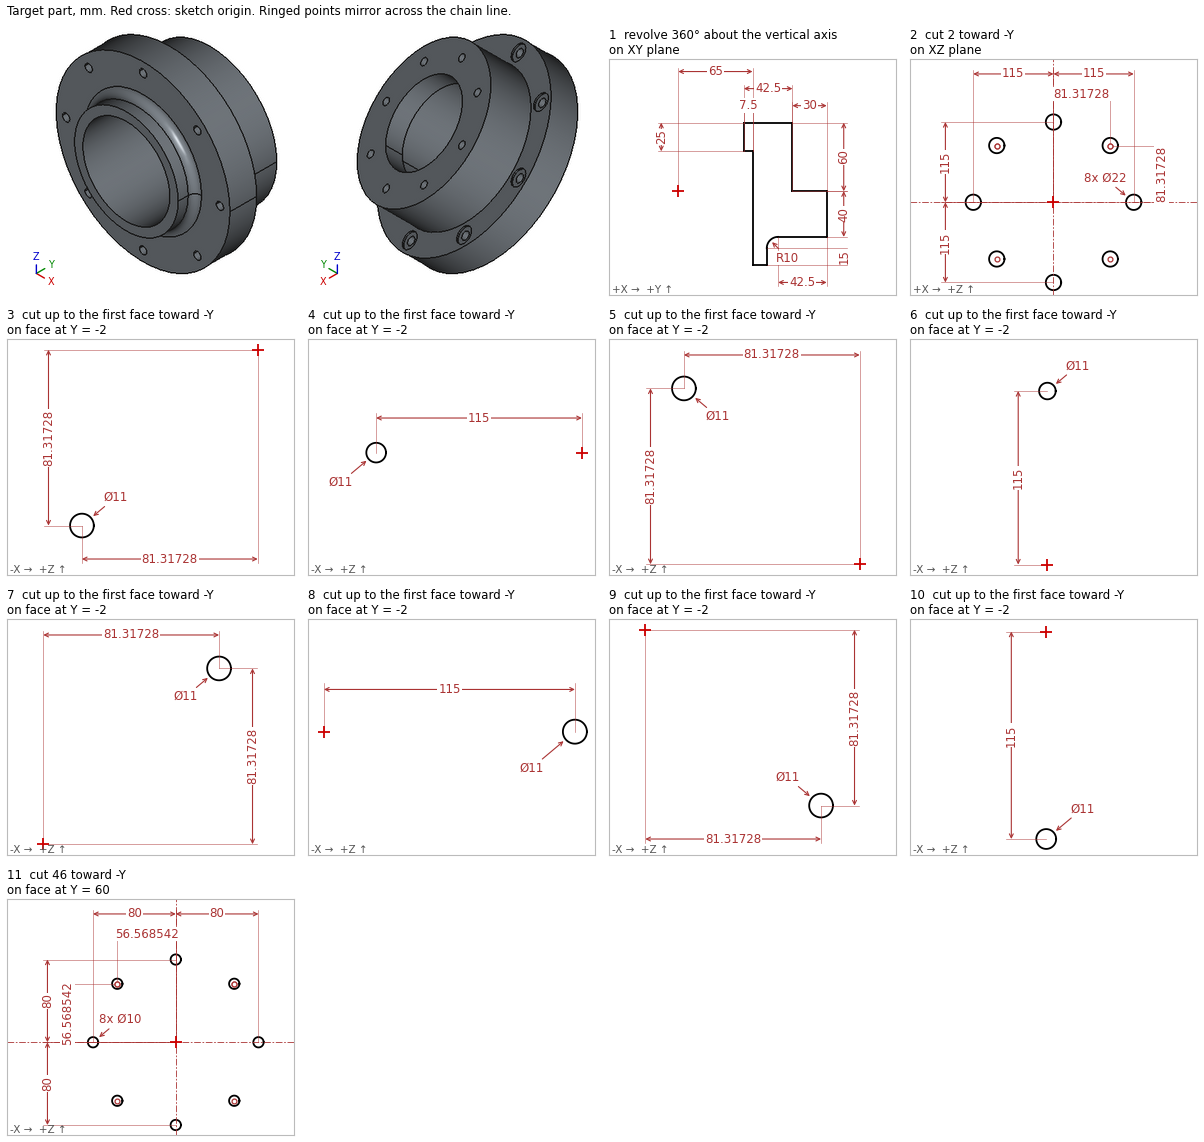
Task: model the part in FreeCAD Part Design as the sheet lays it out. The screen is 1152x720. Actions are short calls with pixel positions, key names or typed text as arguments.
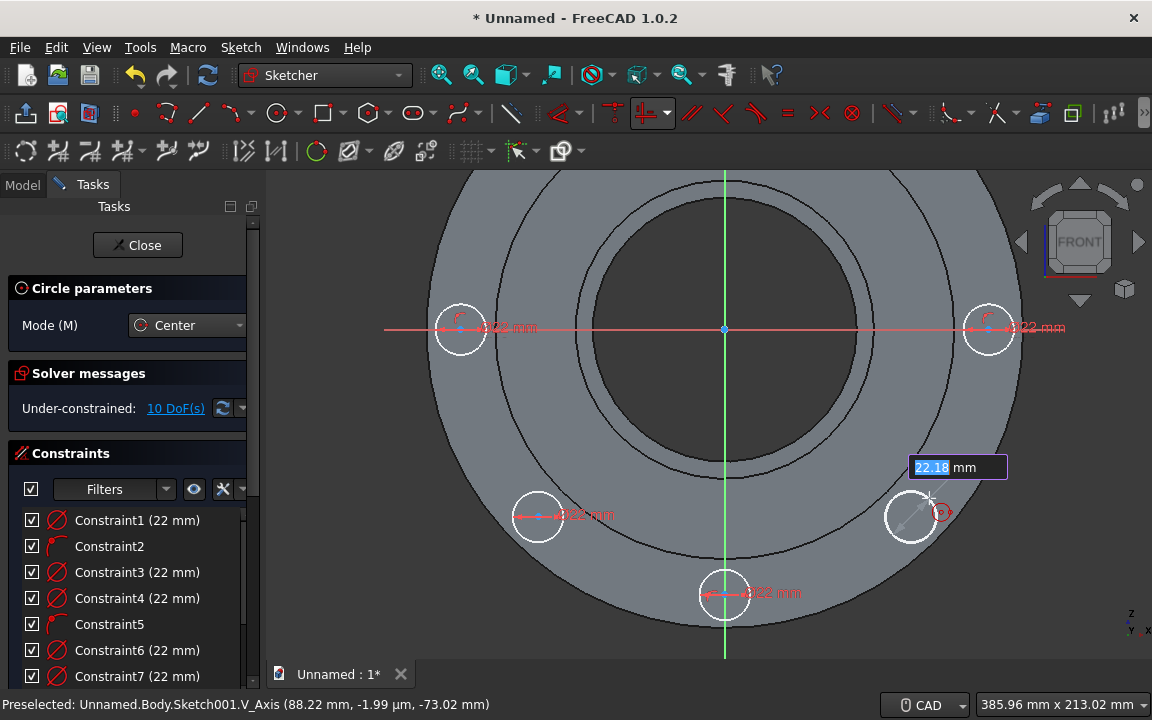
text(22)
key(Return)
key(Escape)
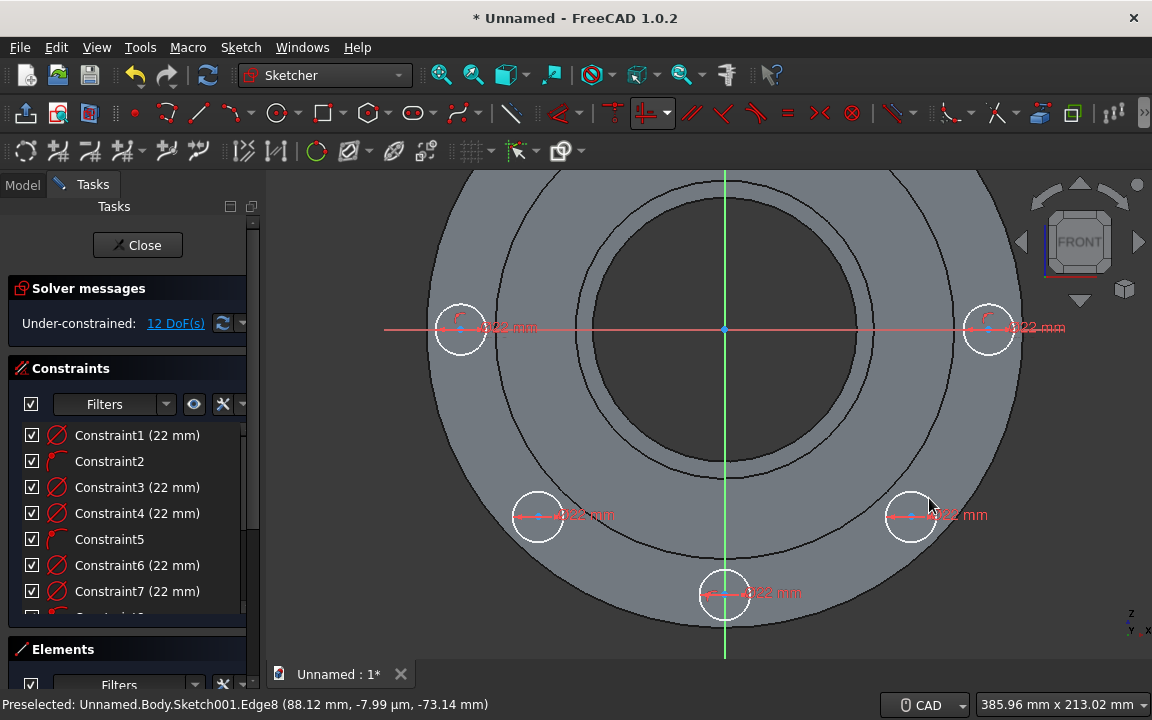
scroll(538, 518, down, 3)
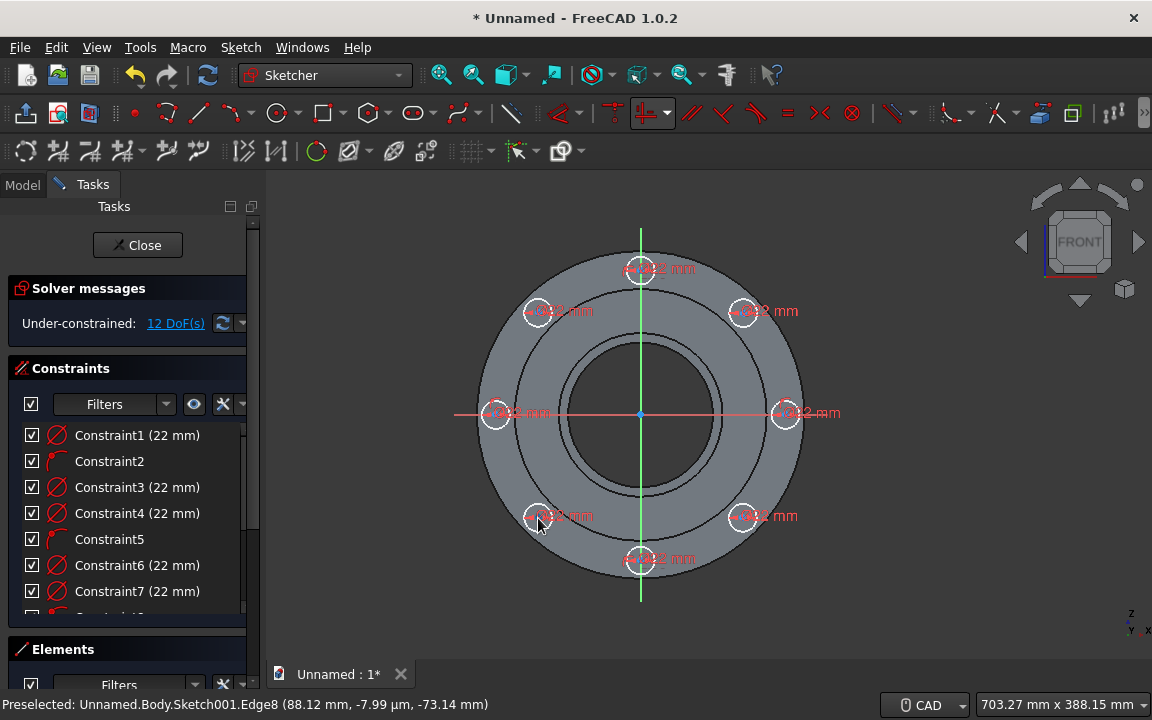
click(743, 313)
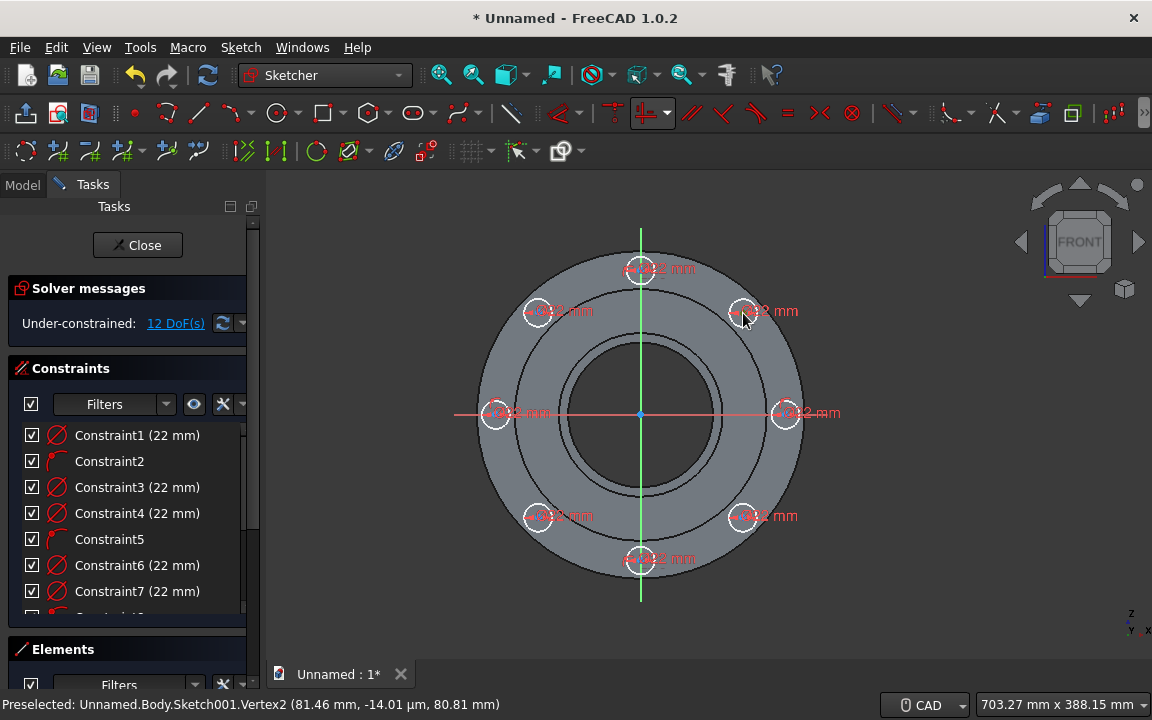
click(538, 313)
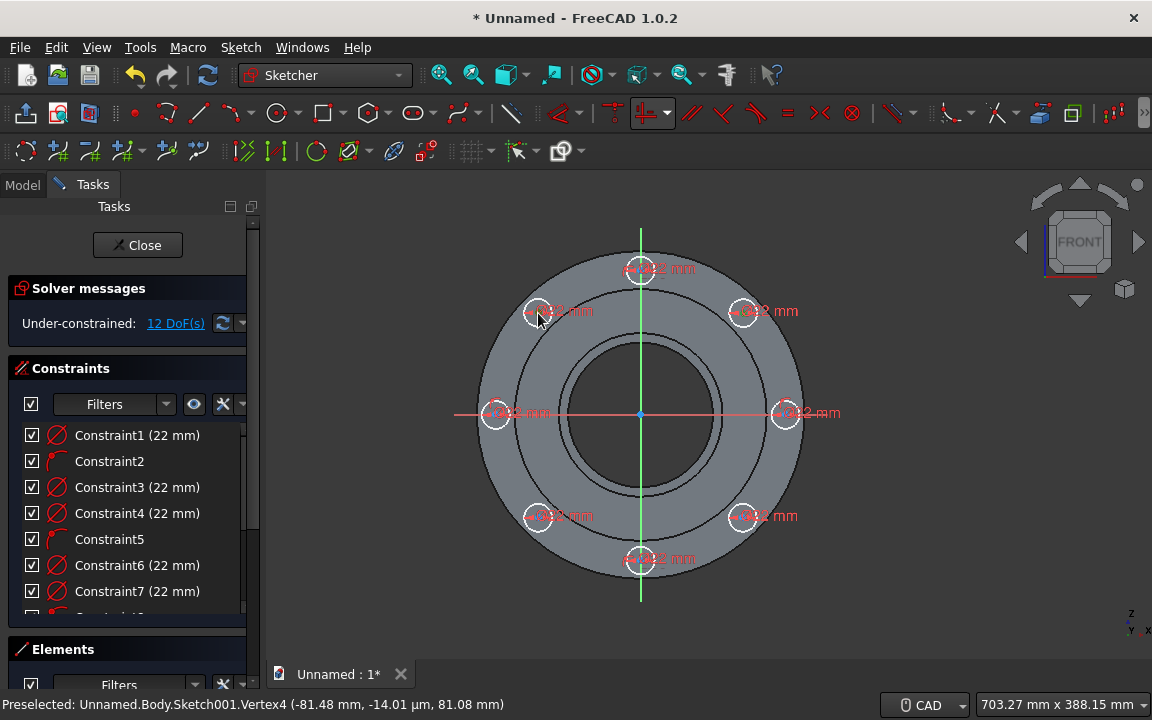
click(641, 507)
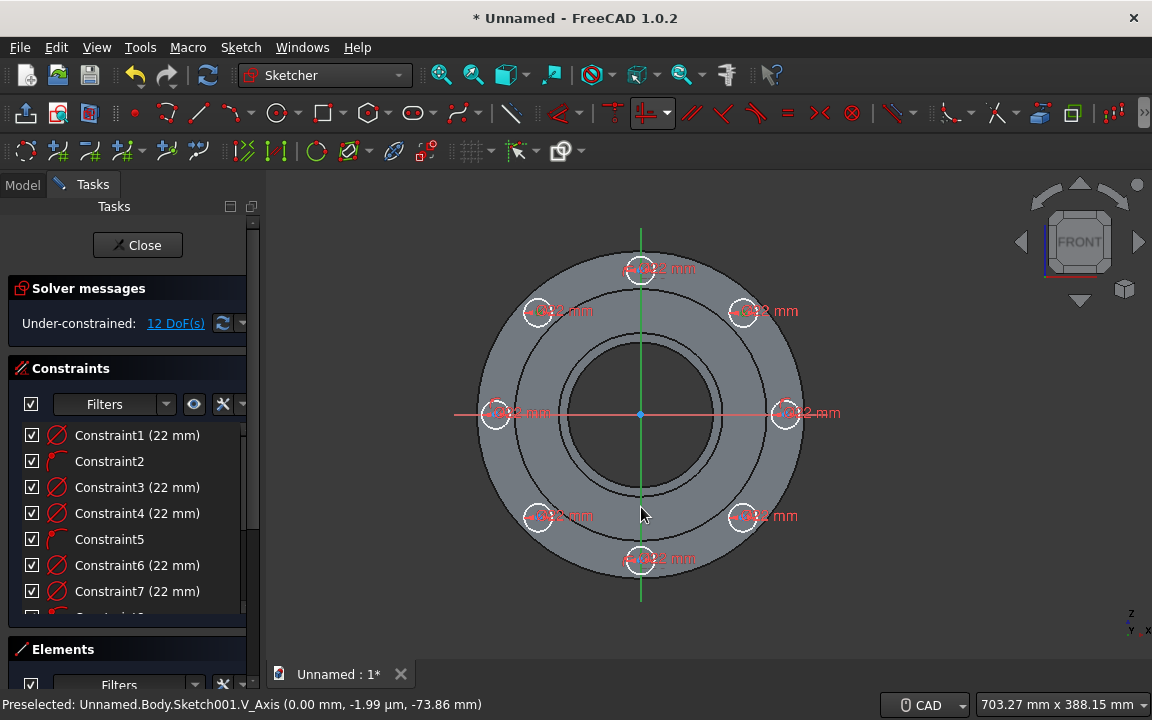
key(s)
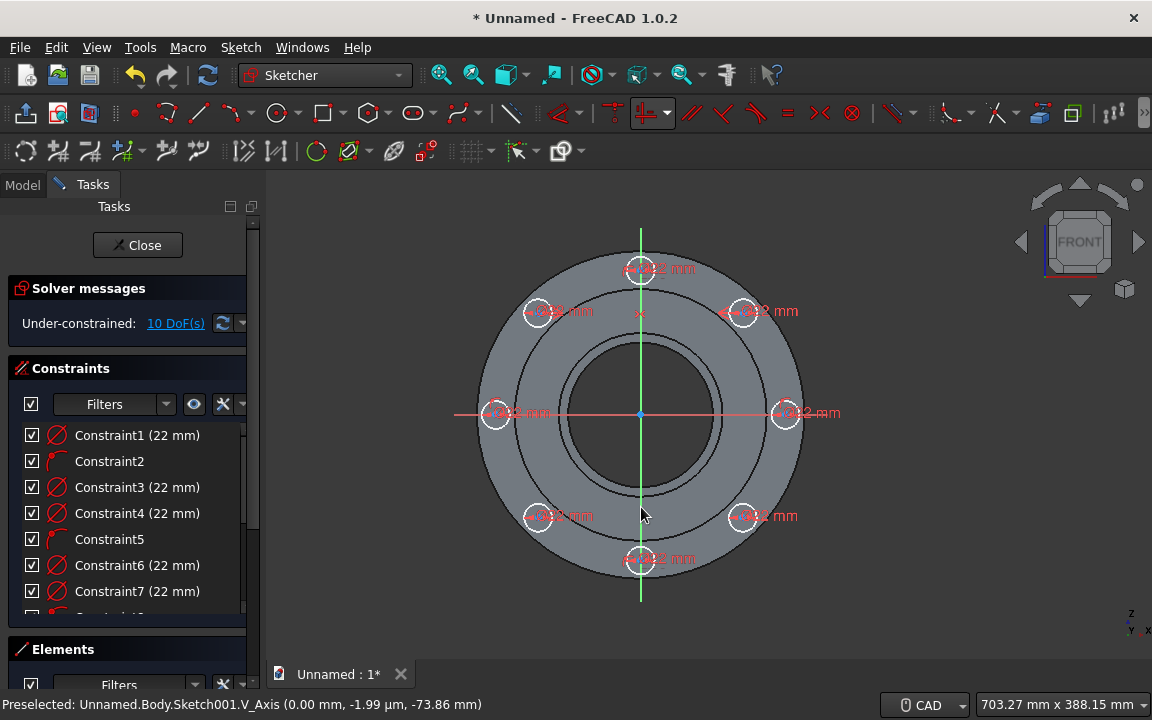
click(538, 313)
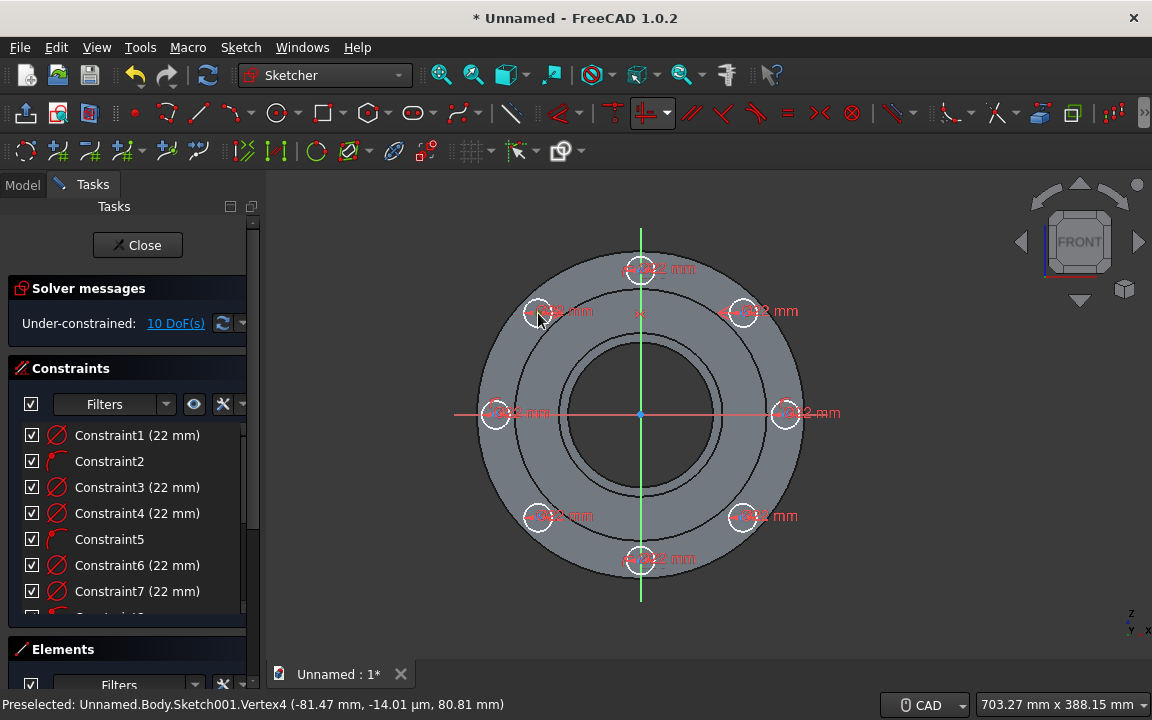
click(538, 518)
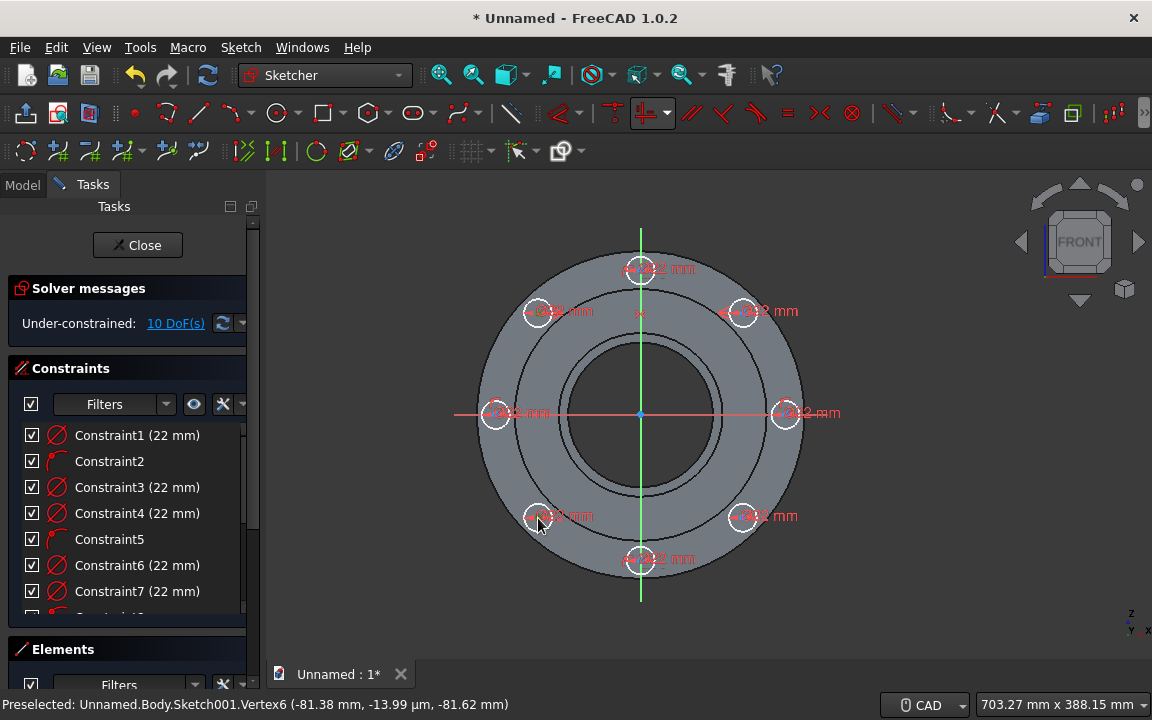
click(591, 415)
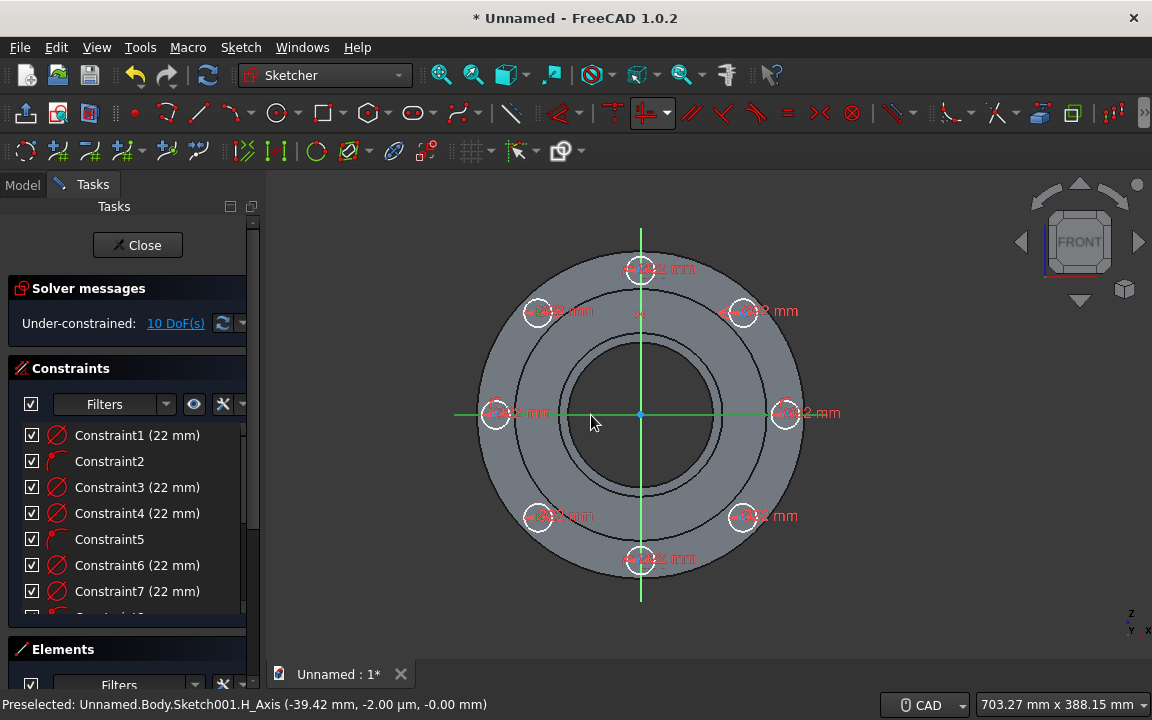
click(820, 114)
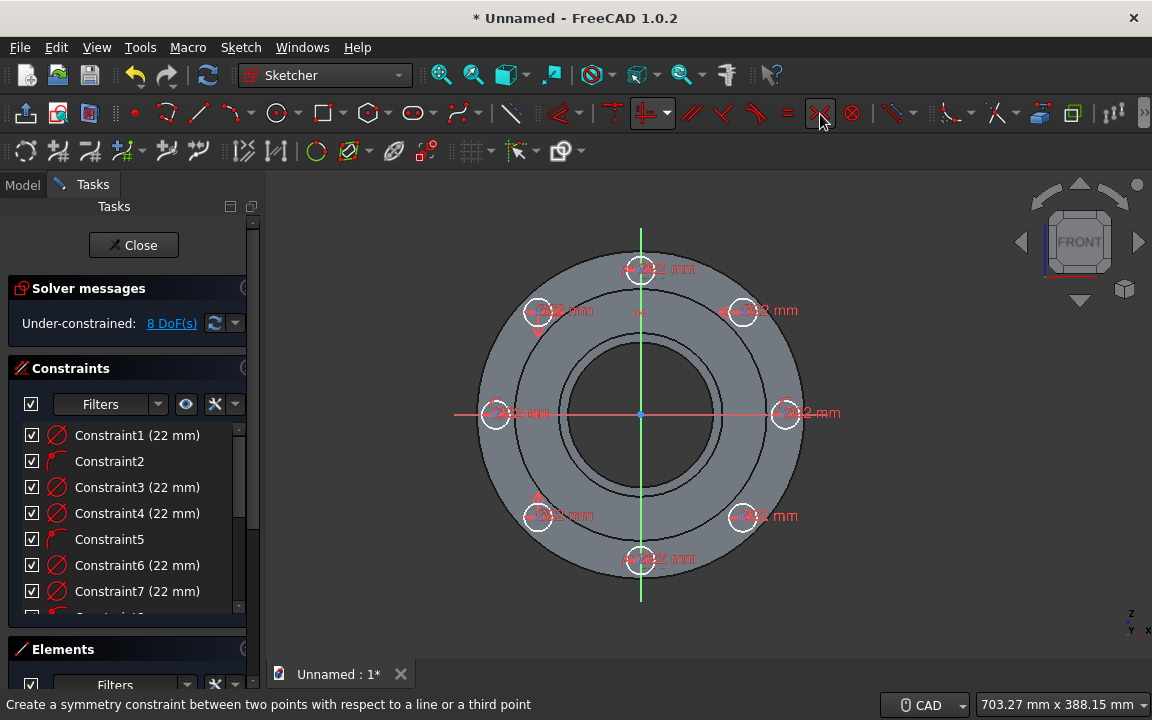
click(743, 312)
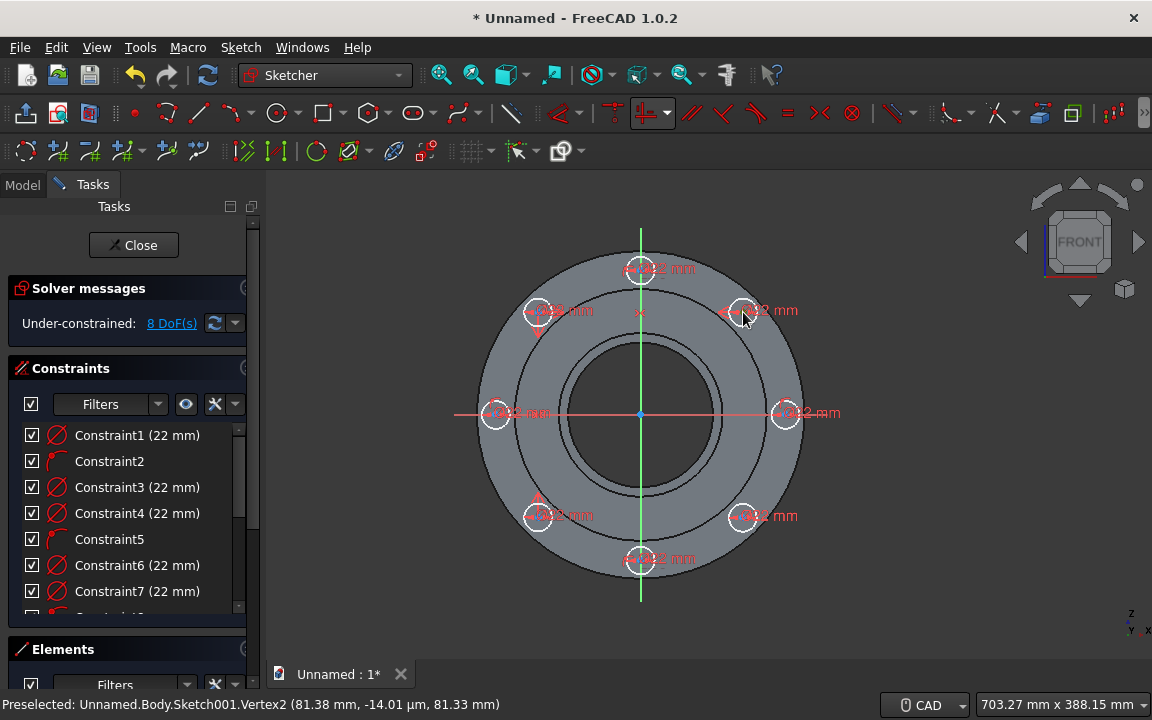
click(743, 518)